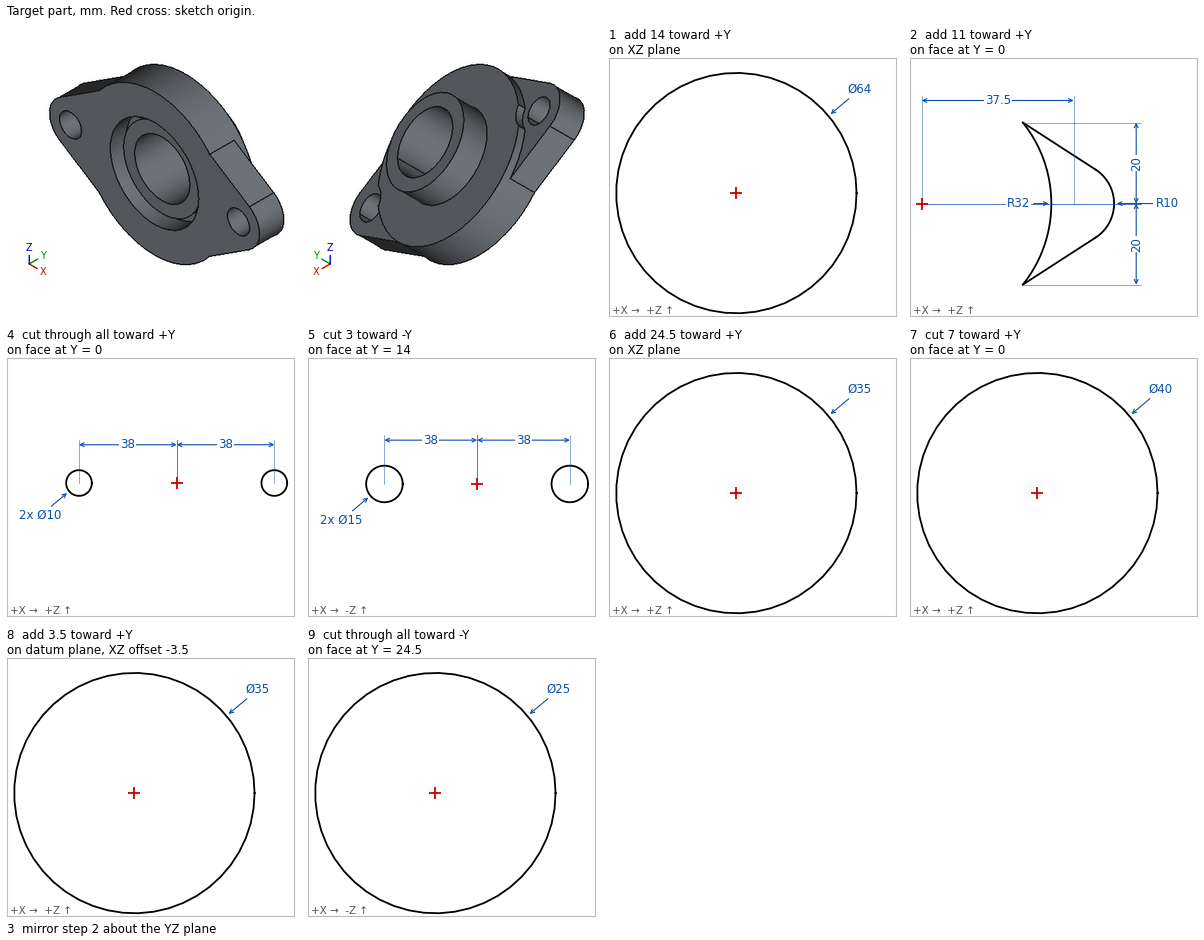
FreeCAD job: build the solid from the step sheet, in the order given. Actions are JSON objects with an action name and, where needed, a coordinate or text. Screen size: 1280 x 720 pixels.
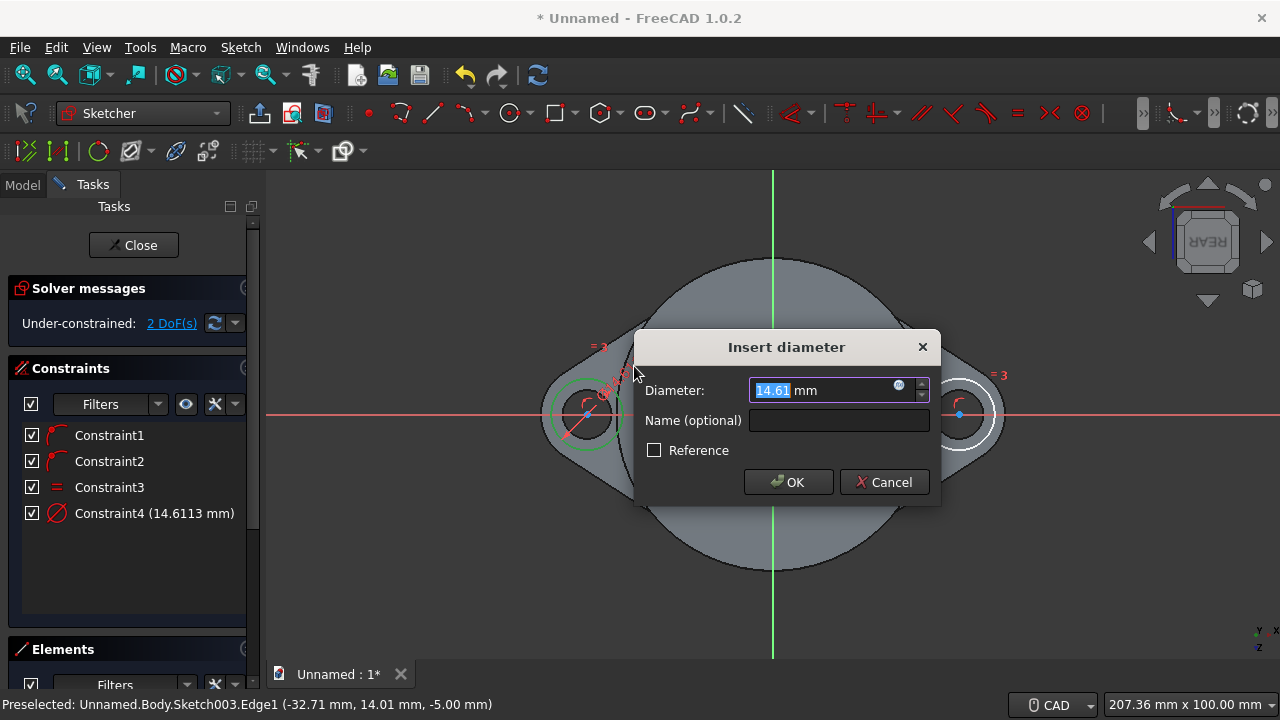
{"action": "type", "text": "15"}
{"action": "key", "text": "Return"}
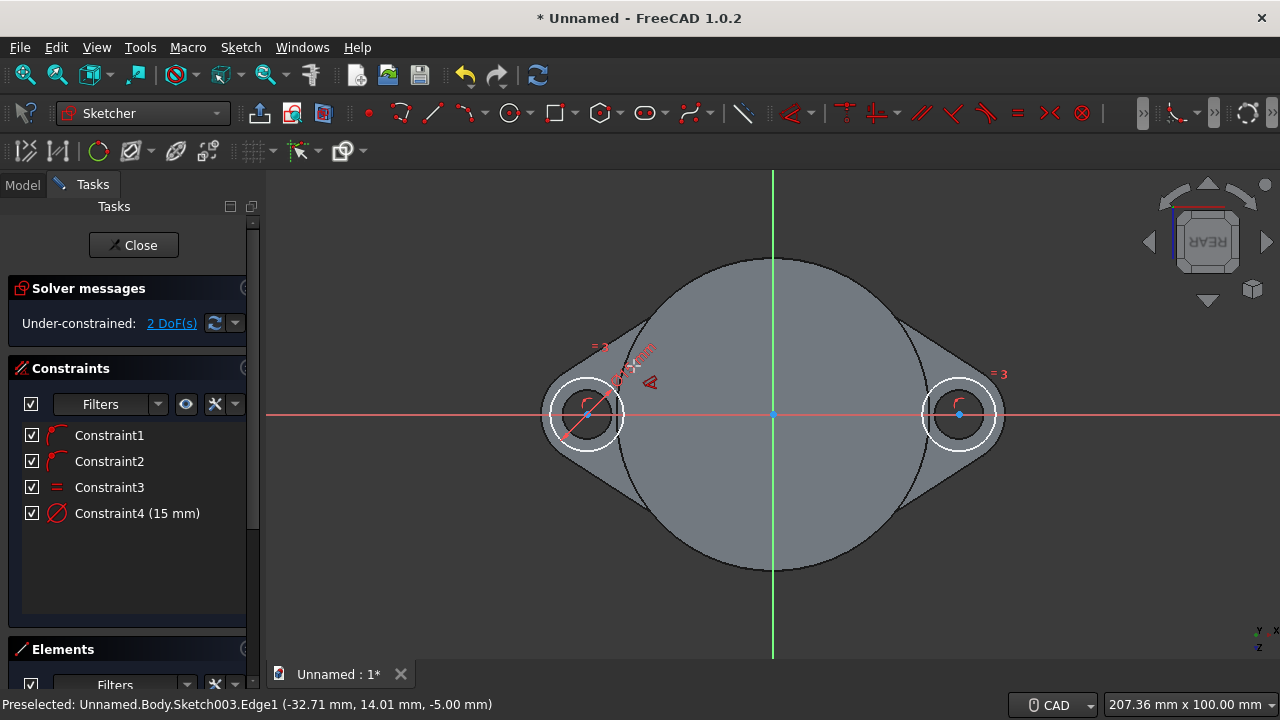
{"action": "left_click", "coordinate": [587, 415]}
{"action": "left_click", "coordinate": [680, 449]}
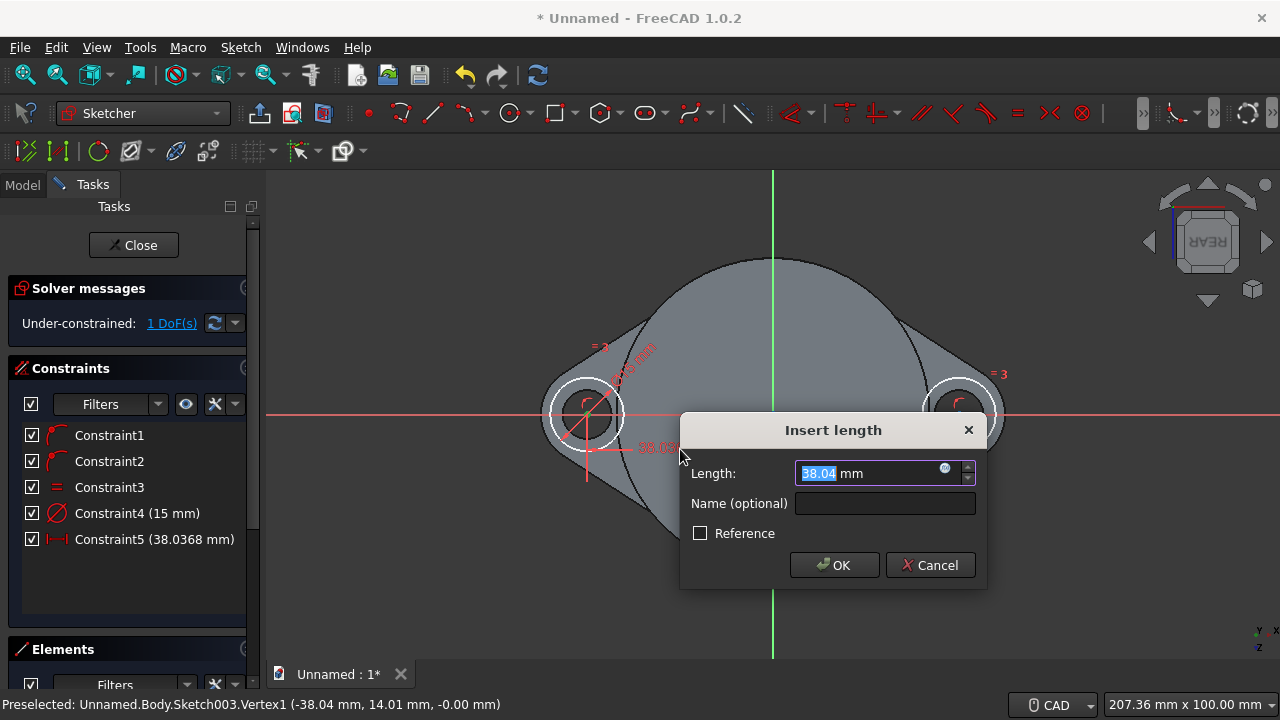
{"action": "type", "text": "38"}
{"action": "key", "text": "Return"}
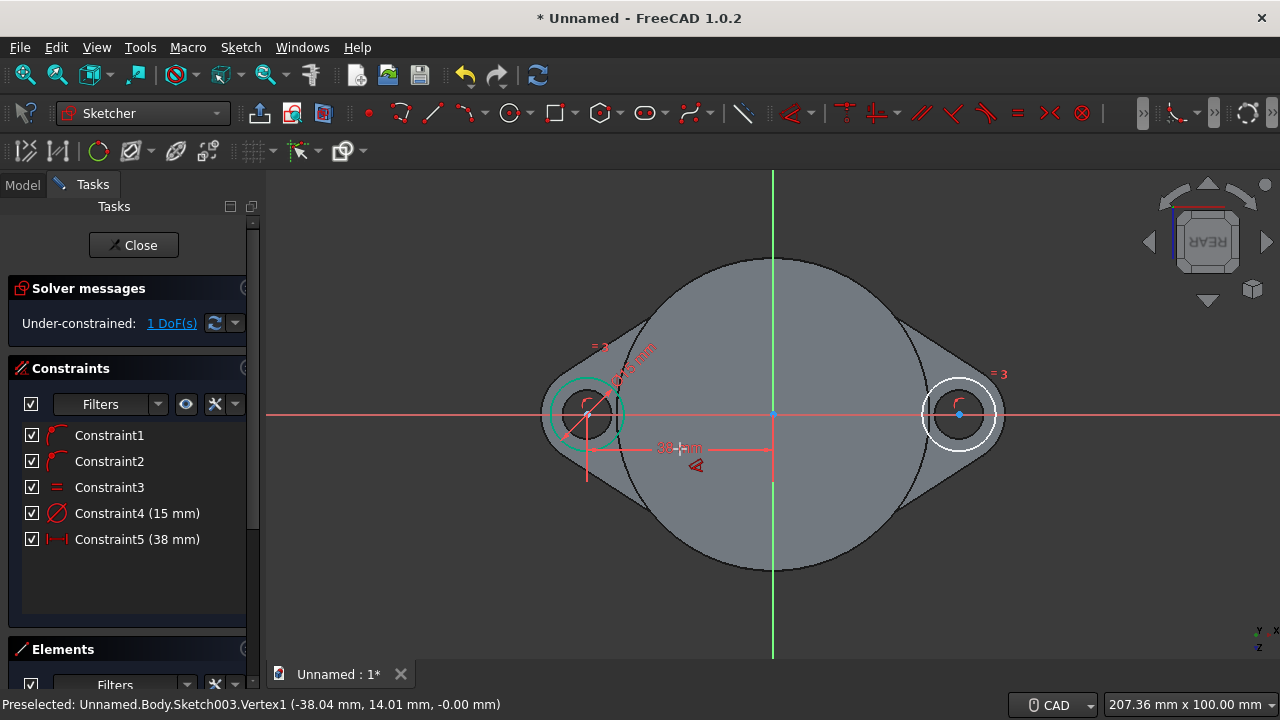
{"action": "left_click", "coordinate": [959, 415]}
{"action": "left_click", "coordinate": [866, 449]}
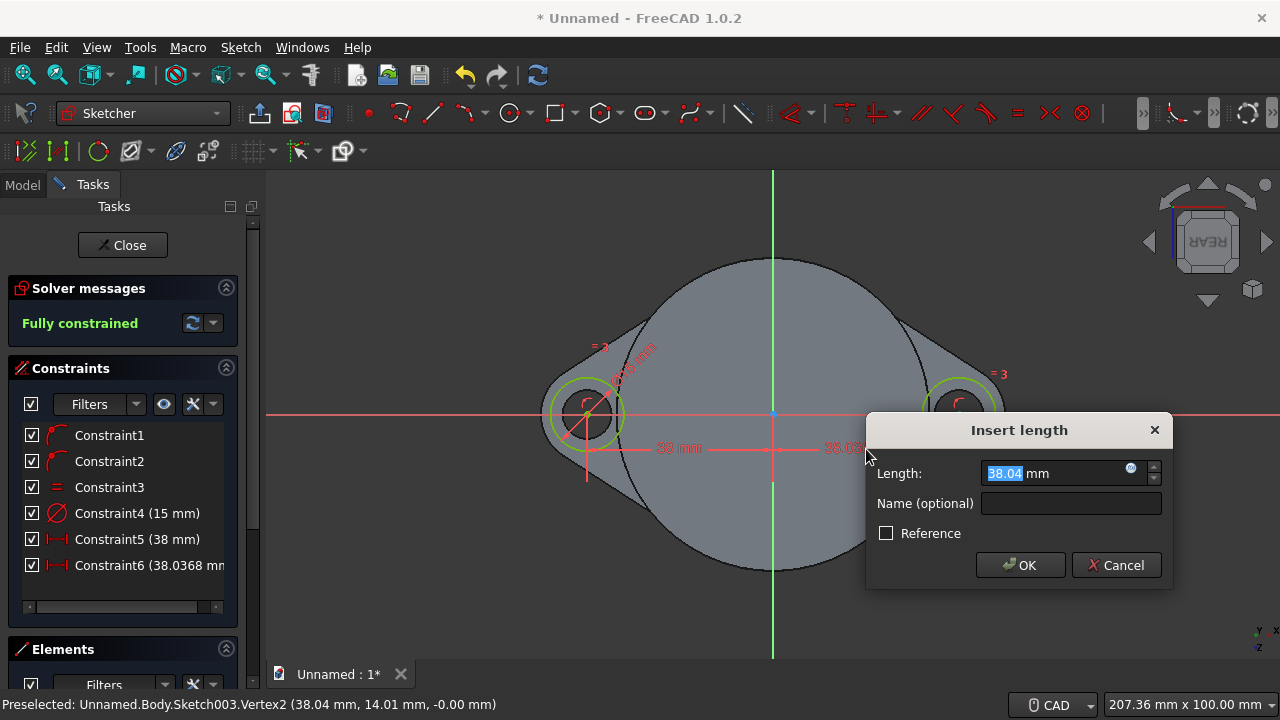
{"action": "type", "text": "38"}
{"action": "key", "text": "Return"}
{"action": "key", "text": "Escape"}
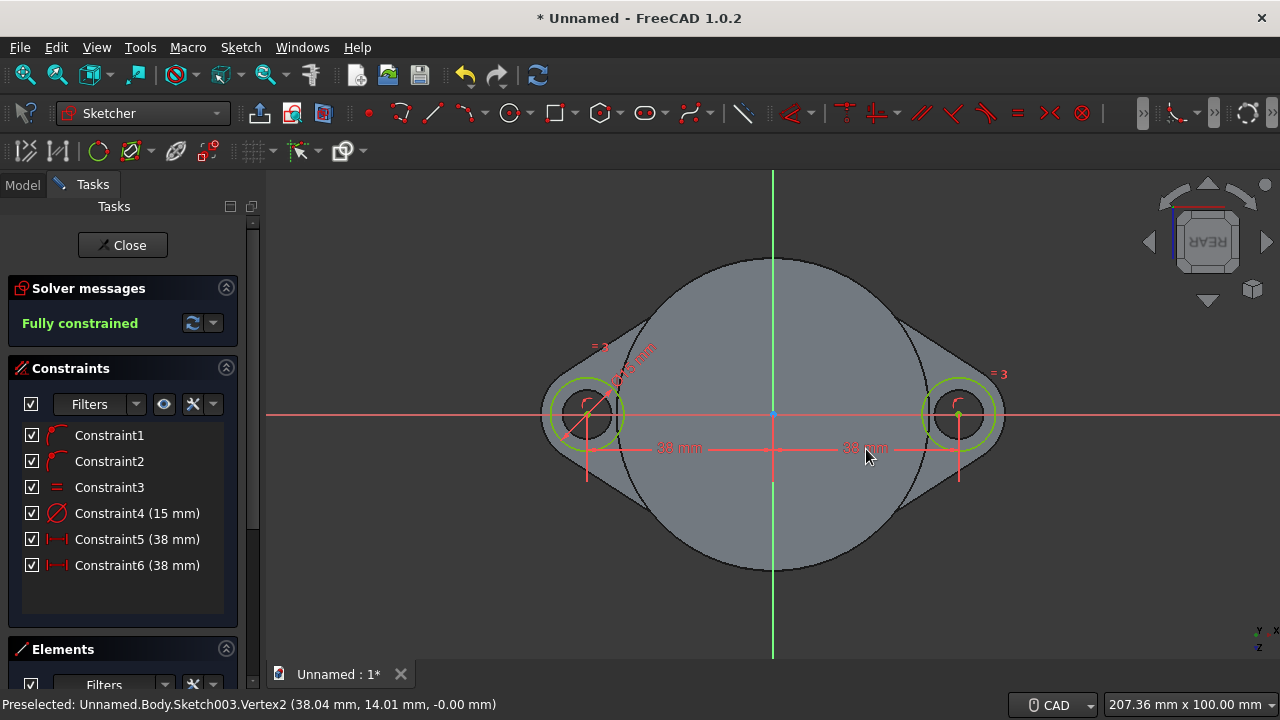
{"action": "left_click", "coordinate": [123, 245]}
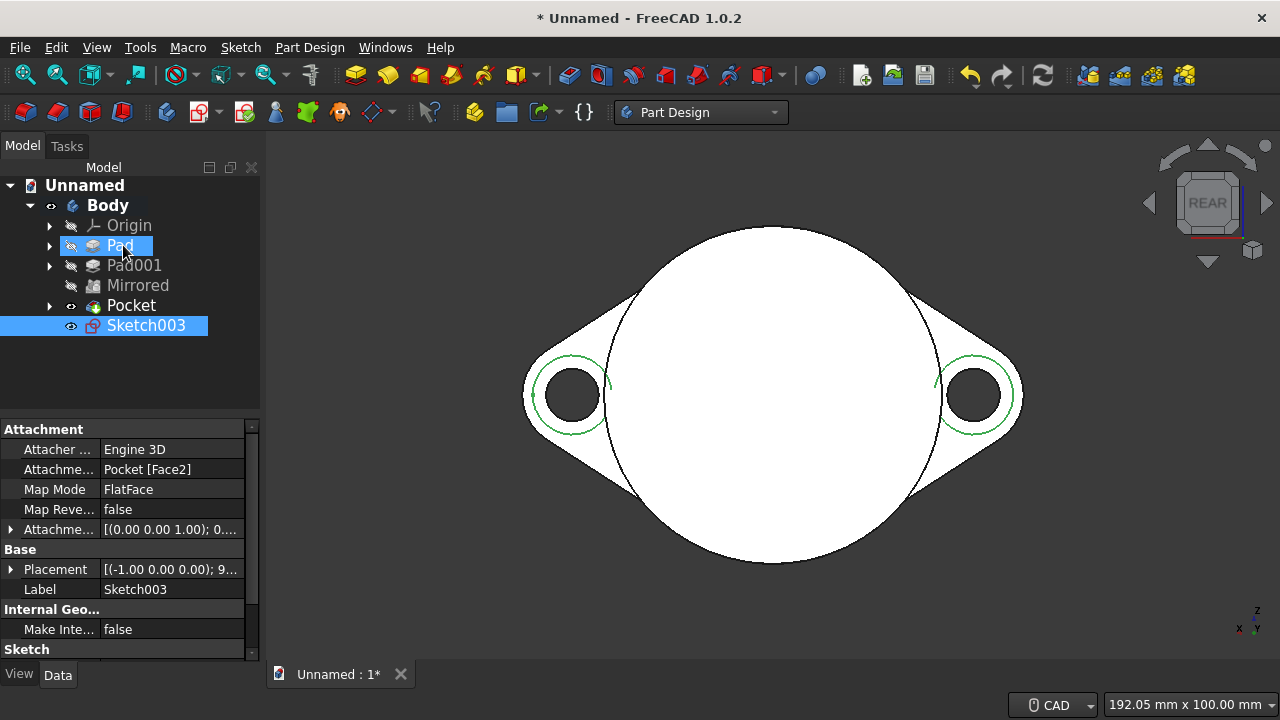
{"action": "left_click", "coordinate": [570, 76]}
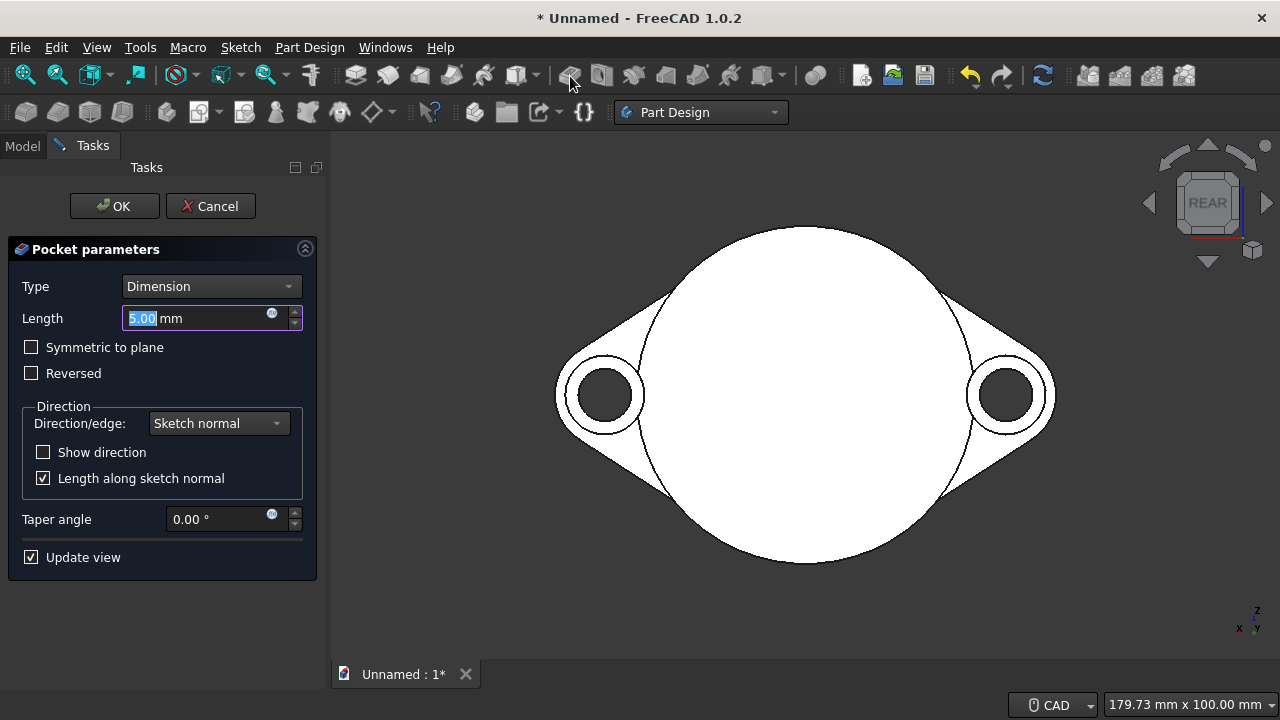
{"action": "type", "text": "3"}
{"action": "key", "text": "Tab"}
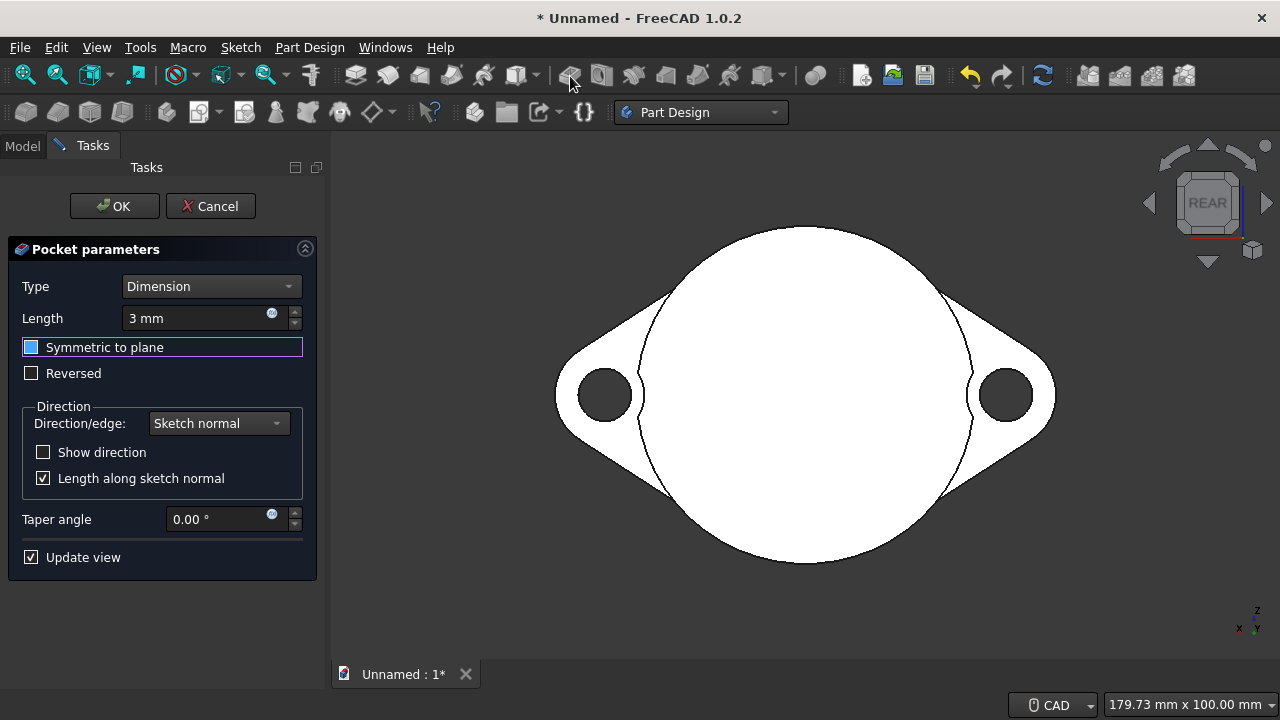
{"action": "left_click", "coordinate": [115, 206]}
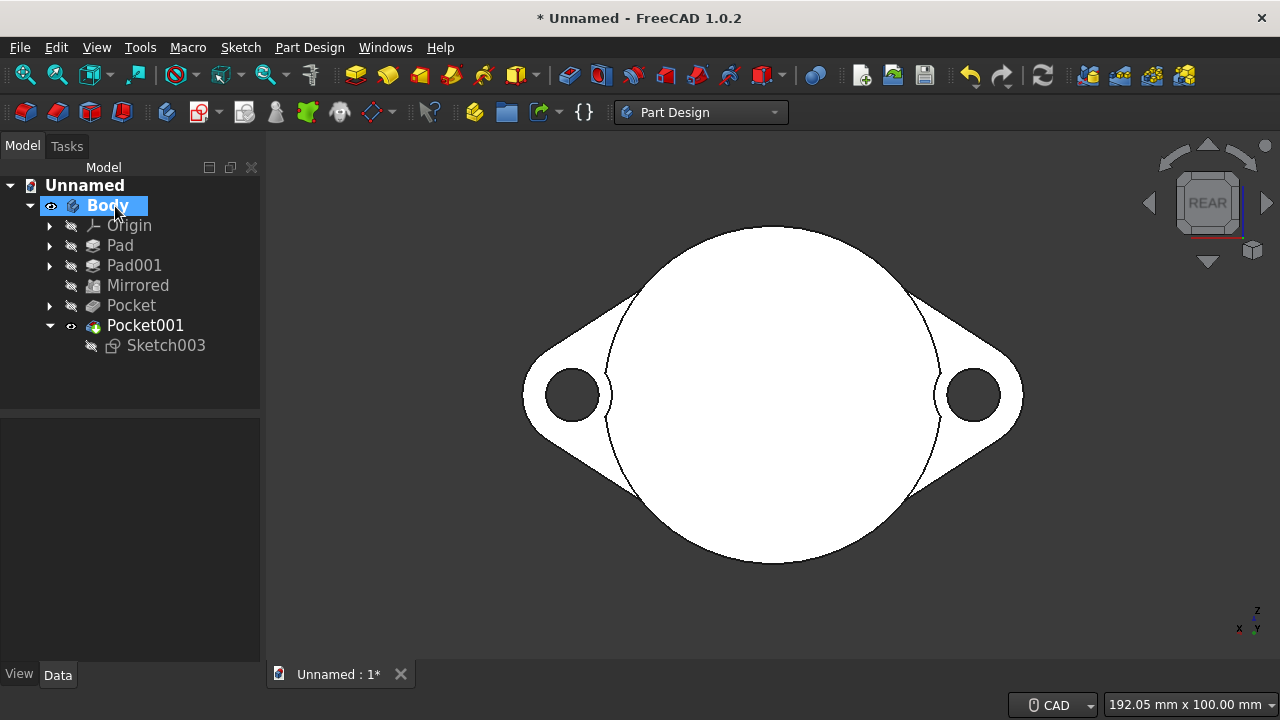
{"action": "left_click", "coordinate": [200, 112]}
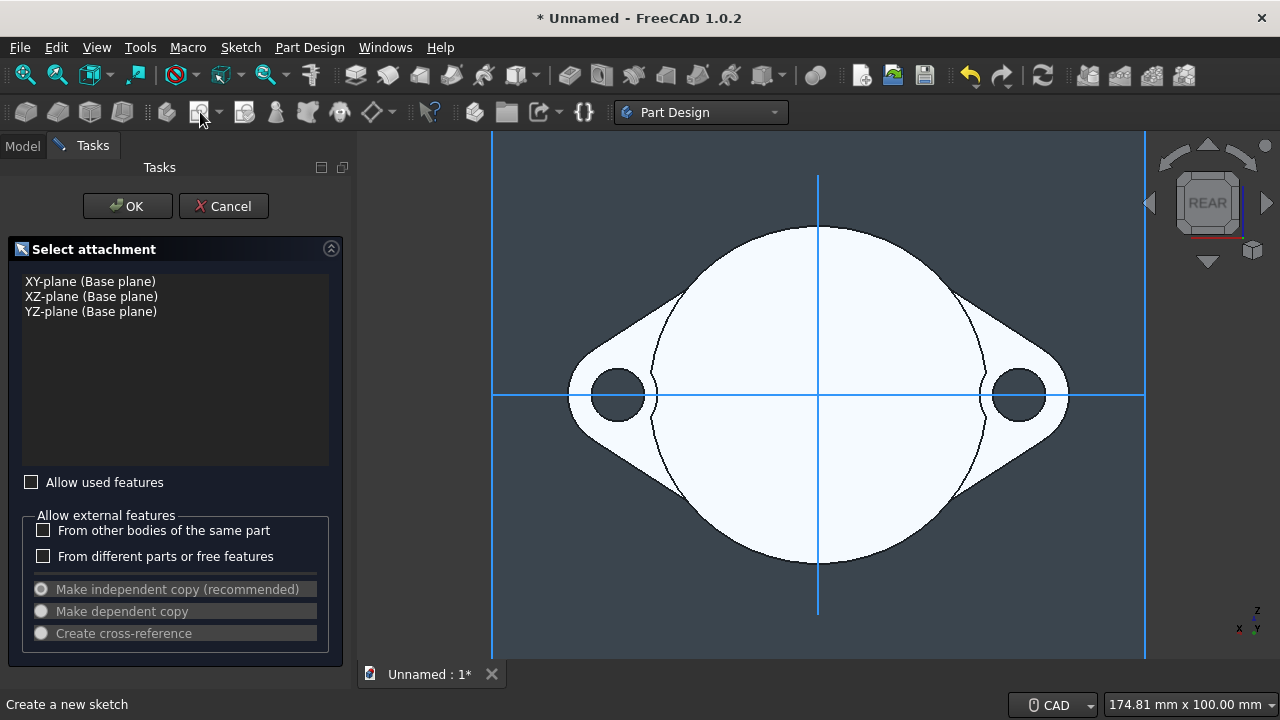
{"action": "left_click", "coordinate": [82, 296]}